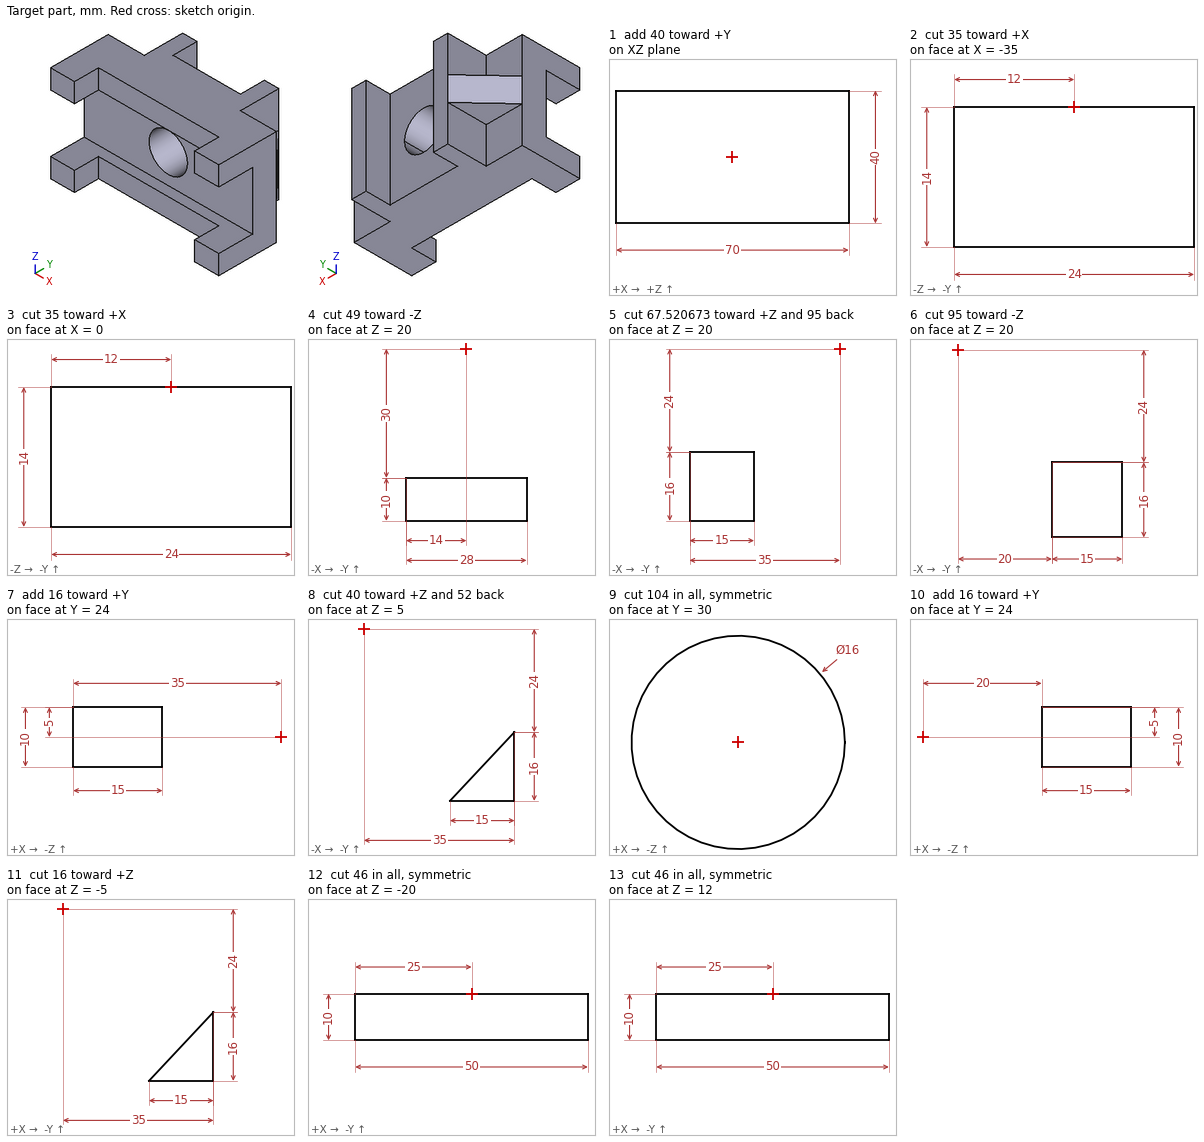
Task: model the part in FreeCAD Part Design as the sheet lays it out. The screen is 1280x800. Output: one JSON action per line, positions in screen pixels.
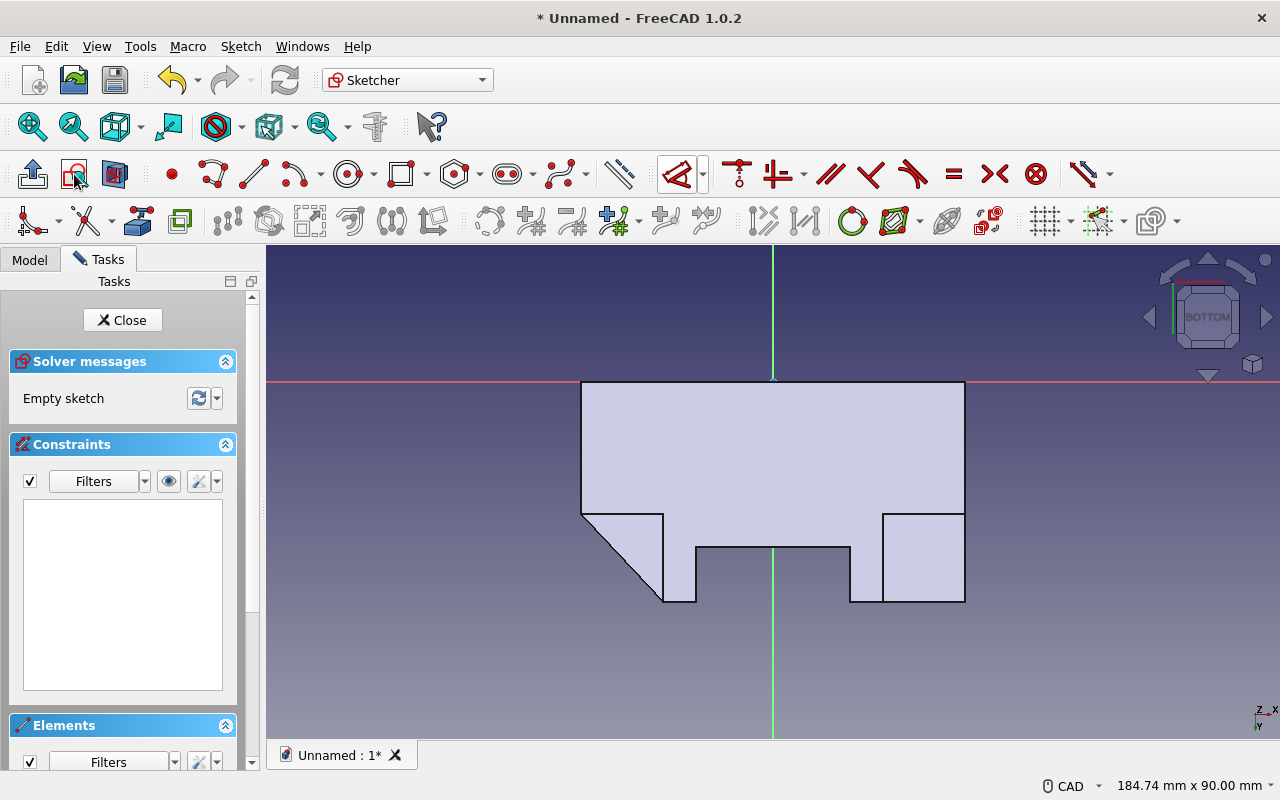
{"action": "scroll", "coordinate": [1019, 586], "scroll_direction": "up", "scroll_amount": 6}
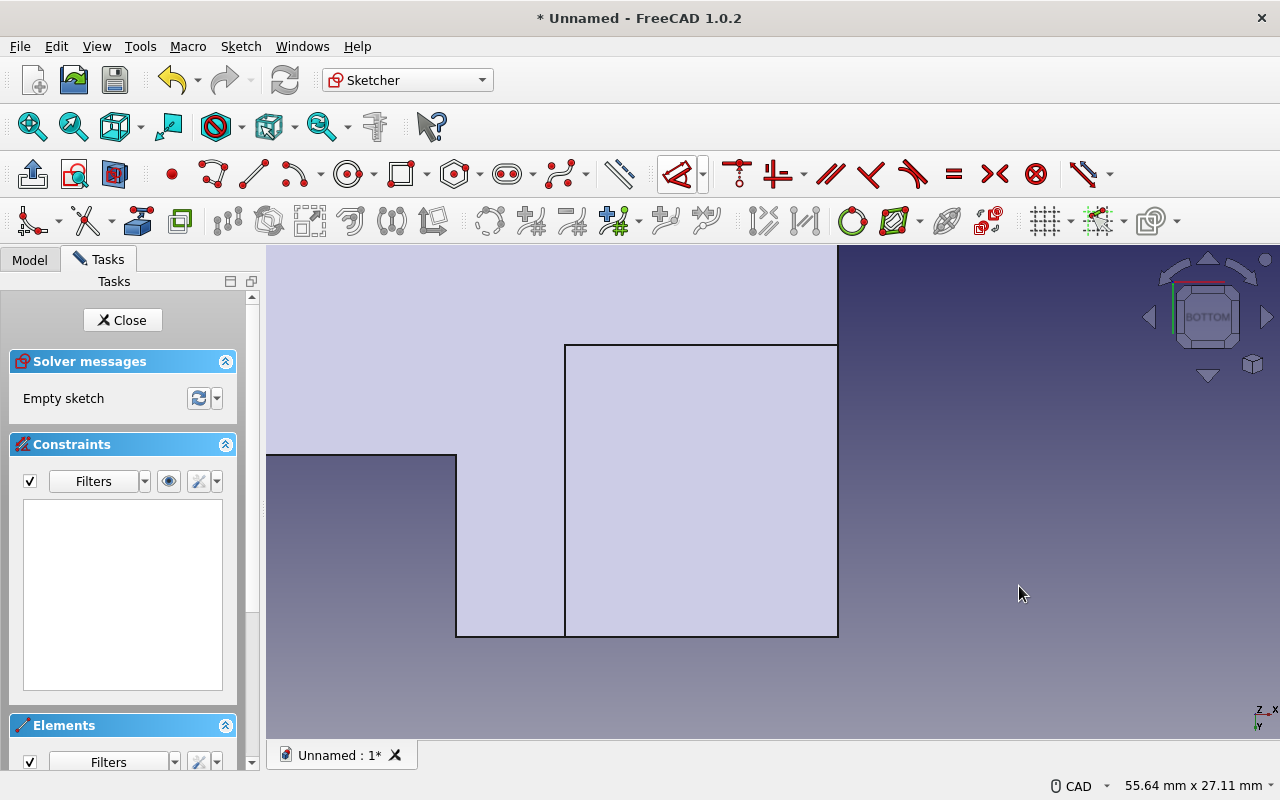
{"action": "left_click", "coordinate": [213, 174]}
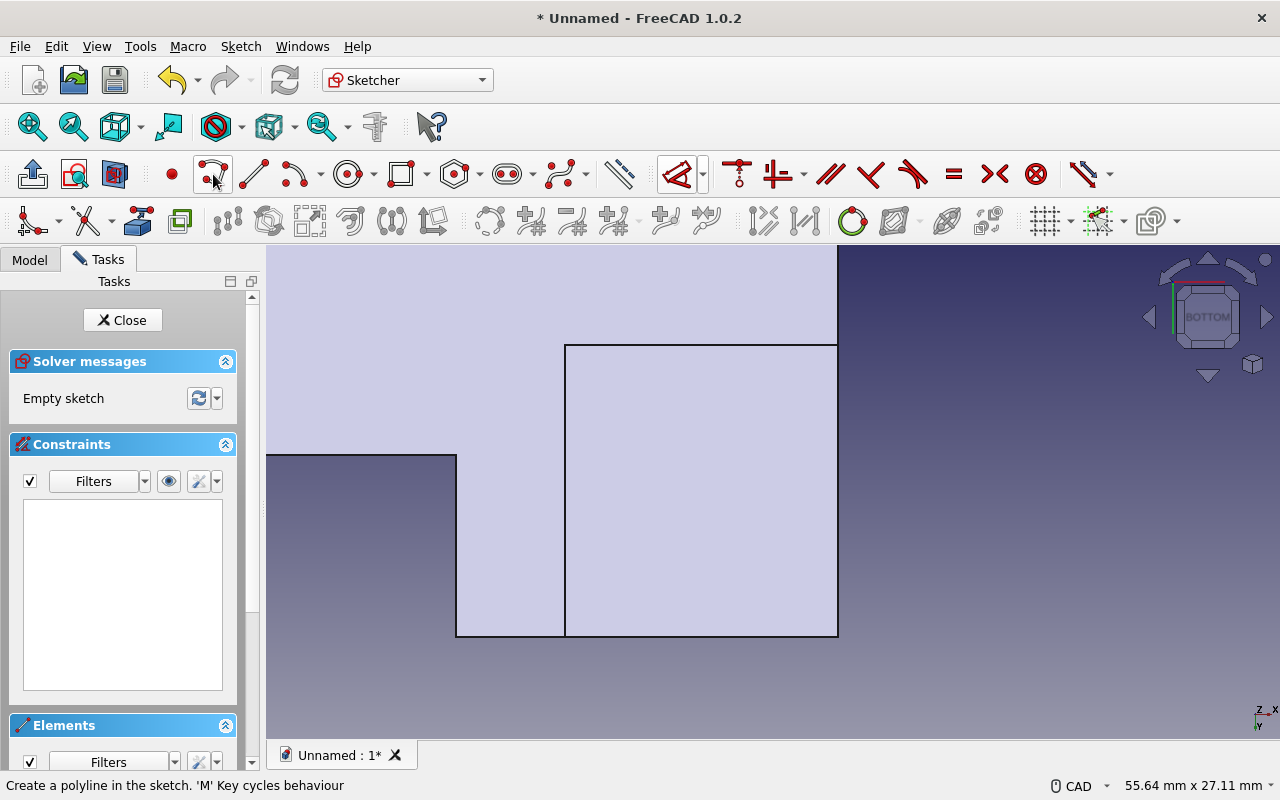
{"action": "left_click", "coordinate": [838, 345]}
{"action": "left_click", "coordinate": [565, 637]}
{"action": "left_click", "coordinate": [838, 637]}
{"action": "left_click", "coordinate": [838, 346]}
{"action": "key", "text": "Escape"}
{"action": "key", "text": "Escape"}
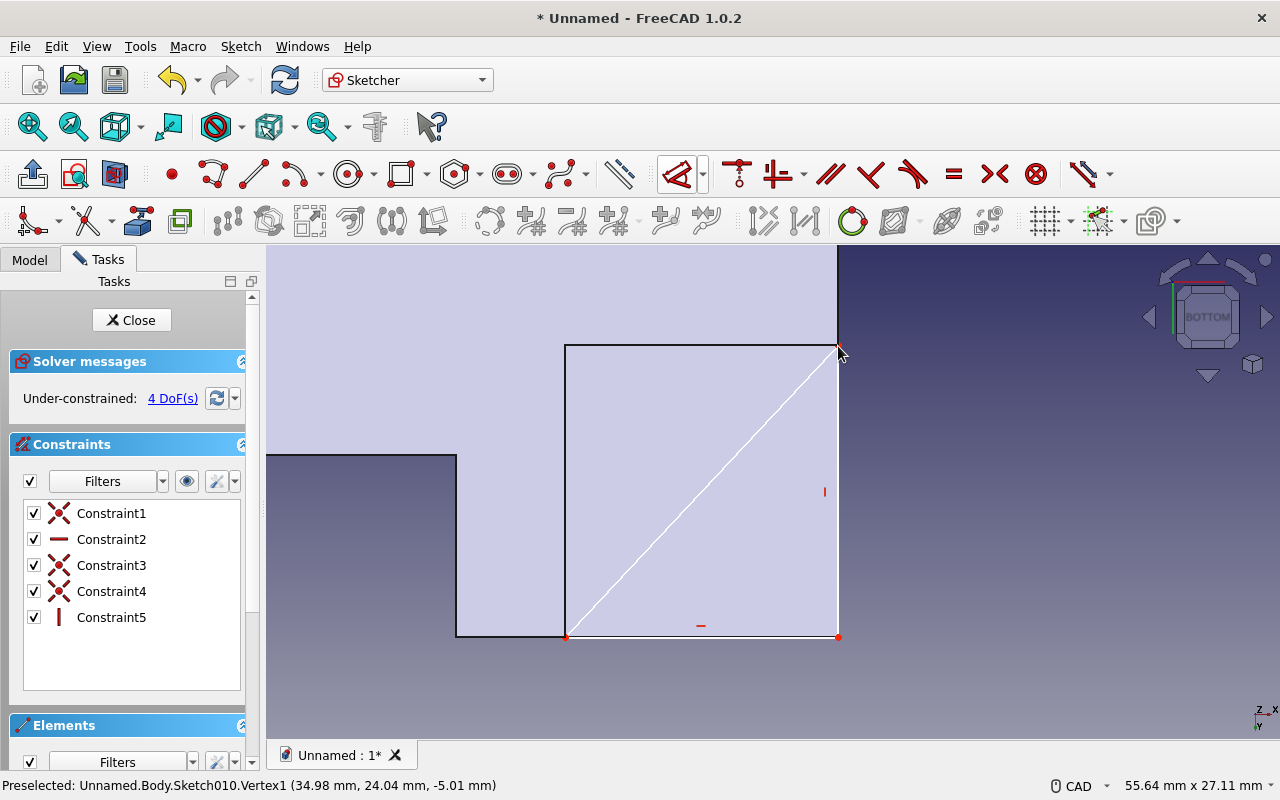
{"action": "left_click", "coordinate": [647, 638]}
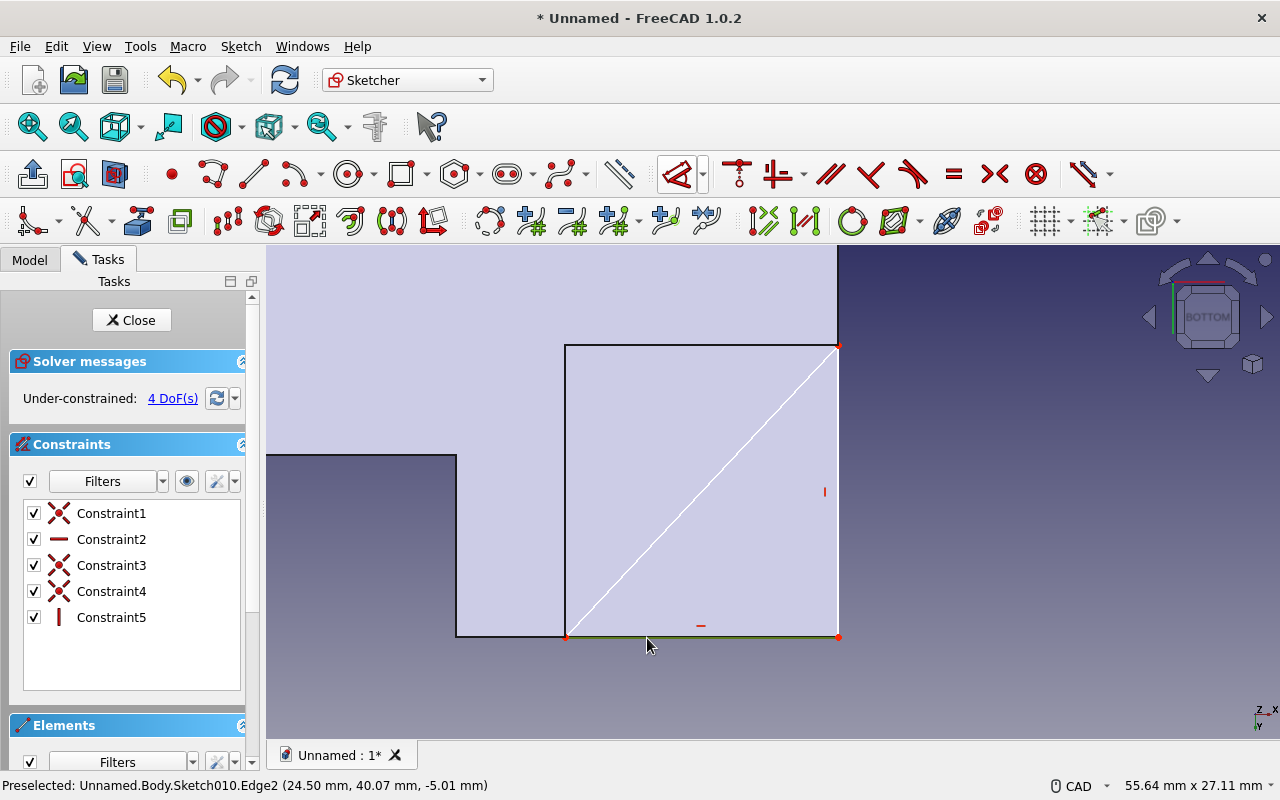
{"action": "key", "text": "l"}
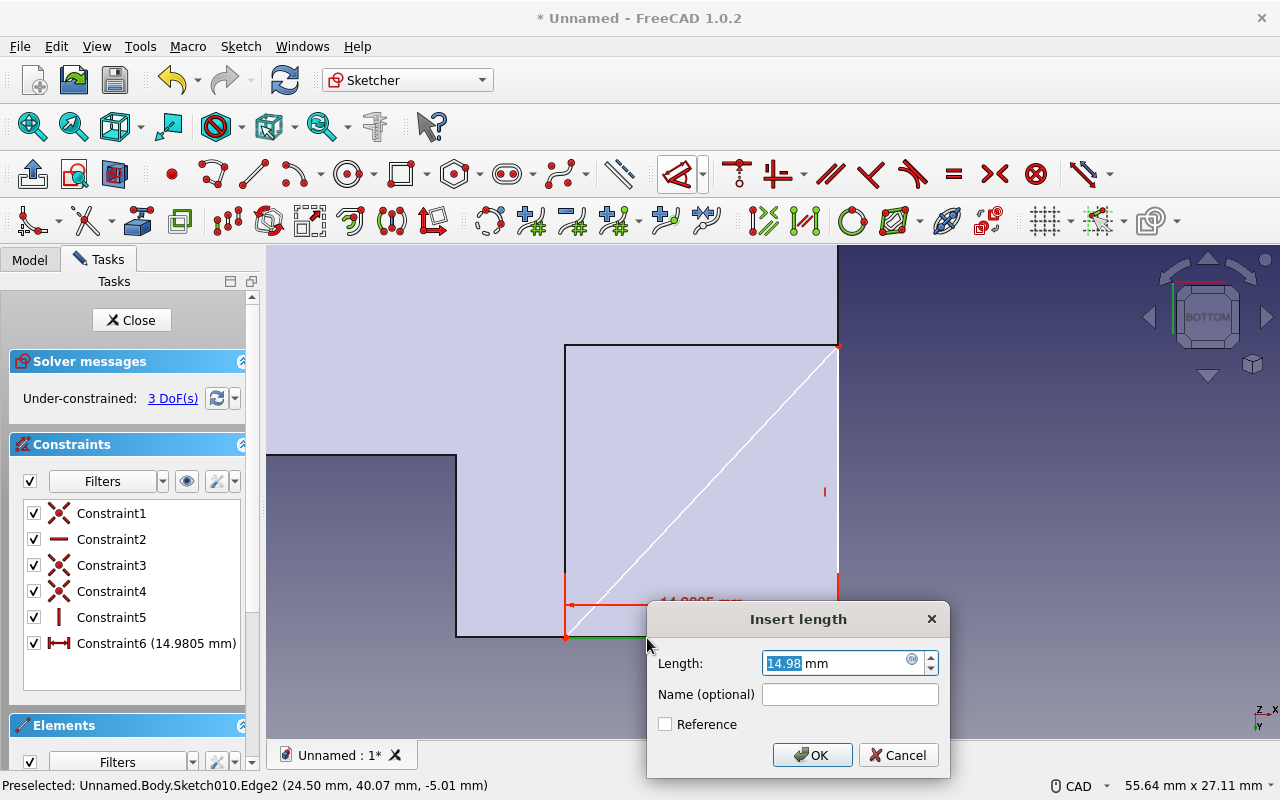
{"action": "type", "text": "15"}
{"action": "key", "text": "Return"}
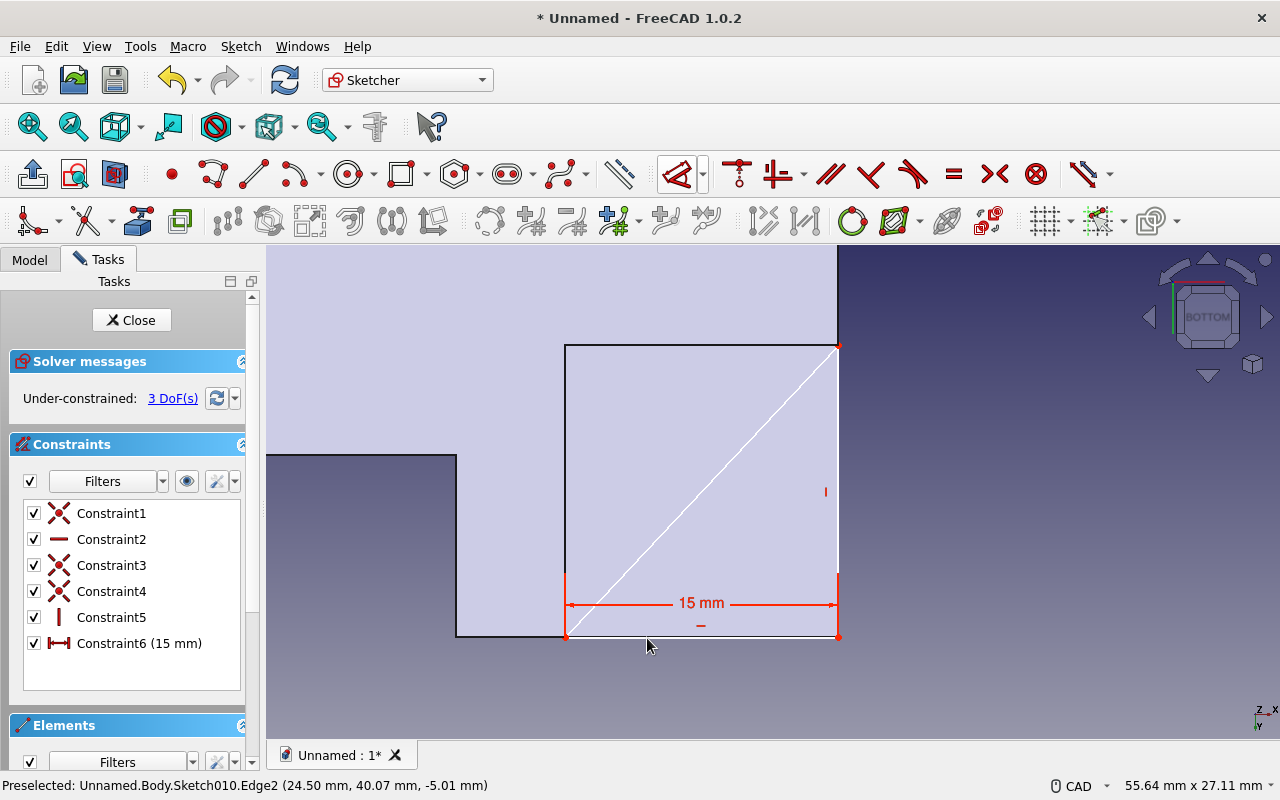
{"action": "left_click", "coordinate": [838, 550]}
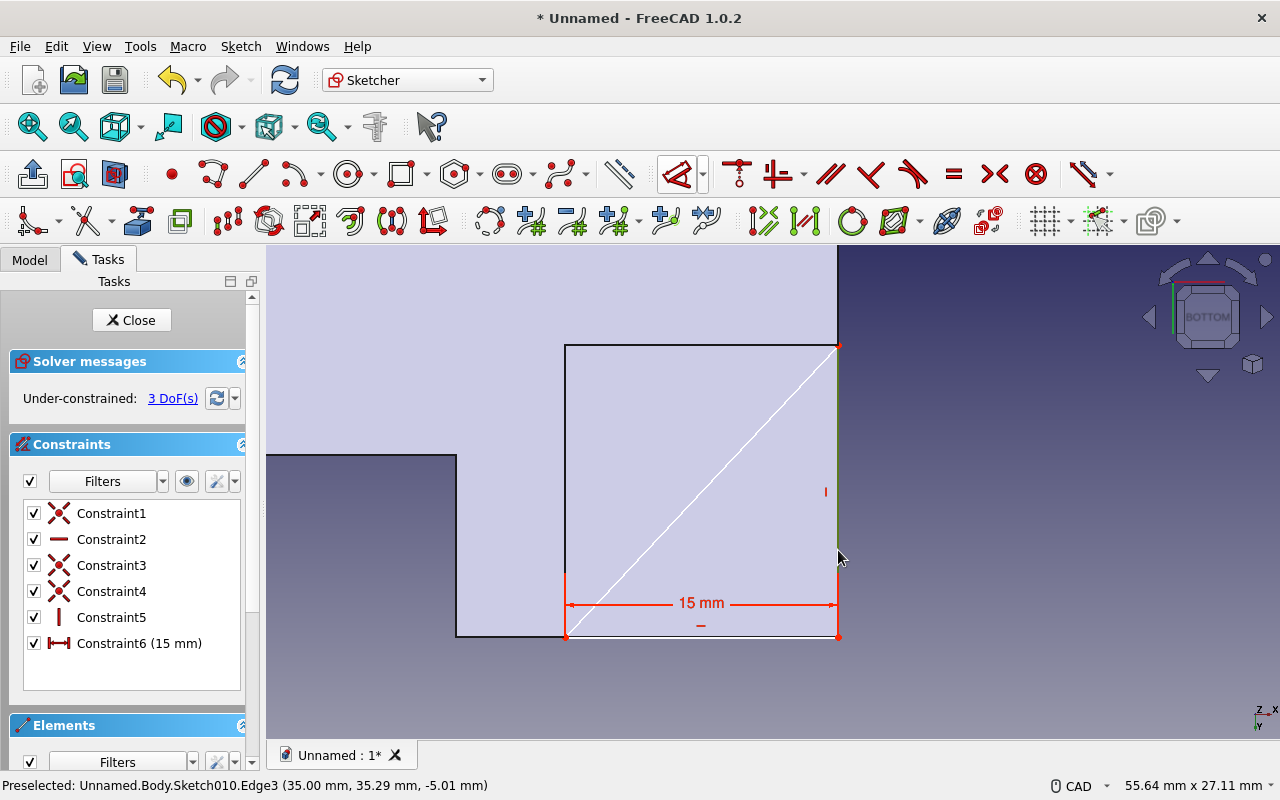
{"action": "key", "text": "i"}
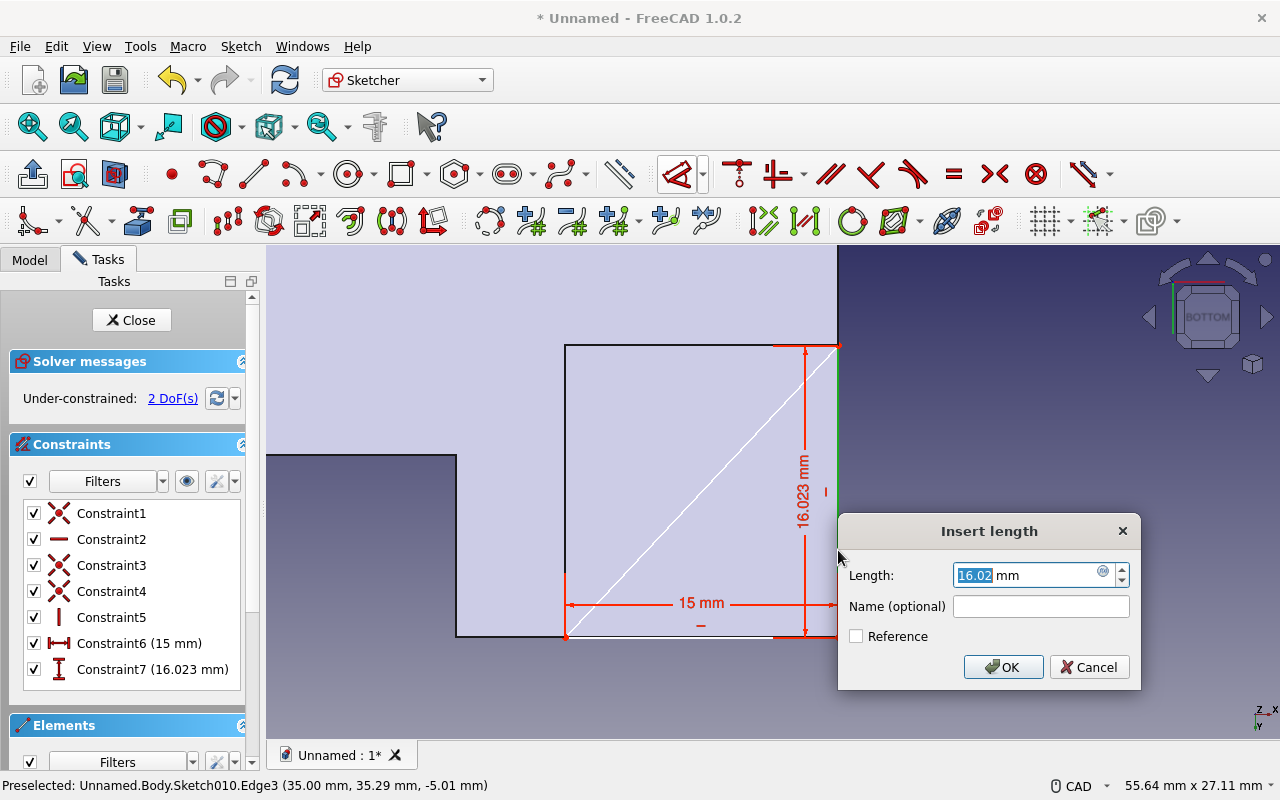
{"action": "type", "text": "16"}
{"action": "key", "text": "Return"}